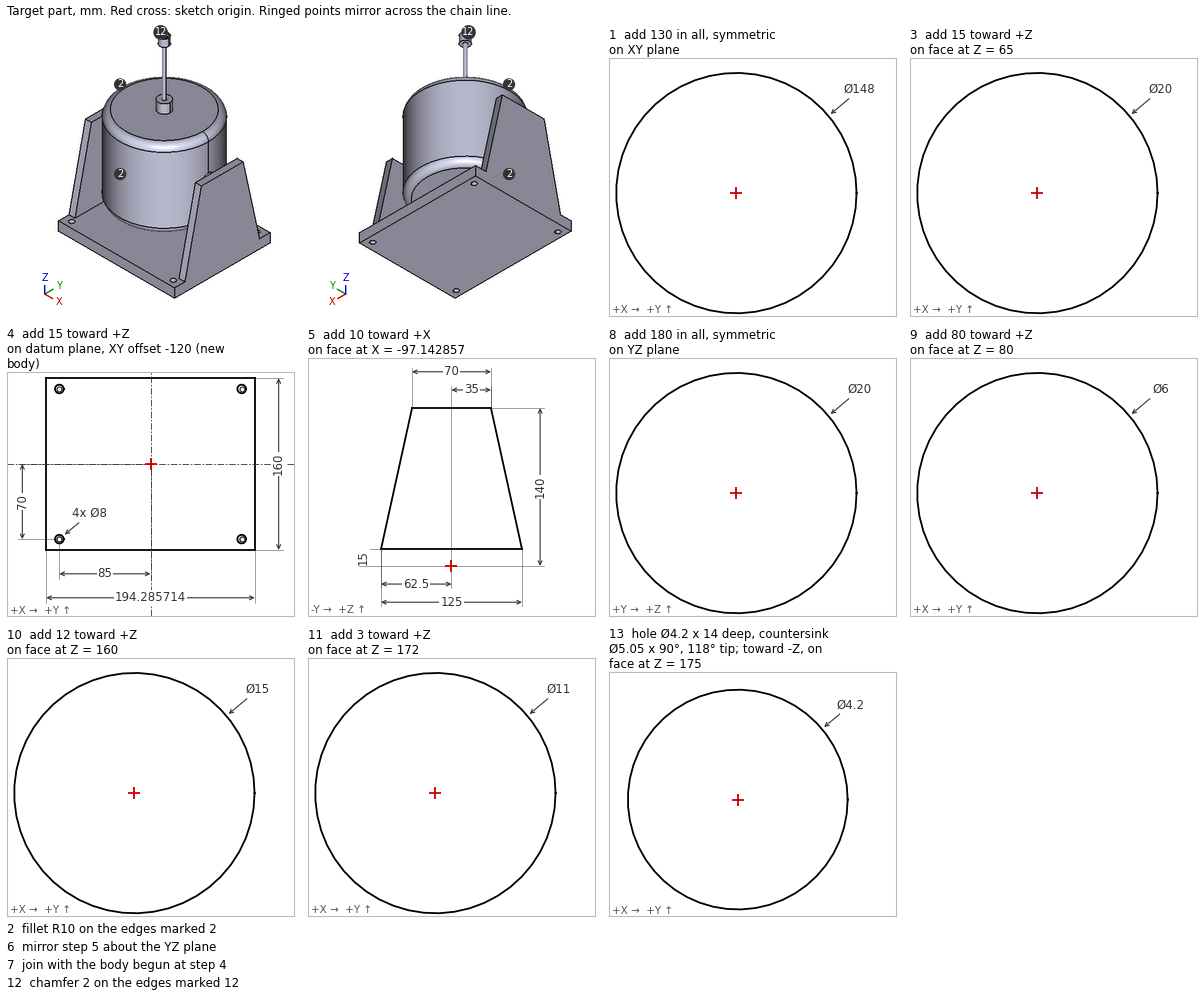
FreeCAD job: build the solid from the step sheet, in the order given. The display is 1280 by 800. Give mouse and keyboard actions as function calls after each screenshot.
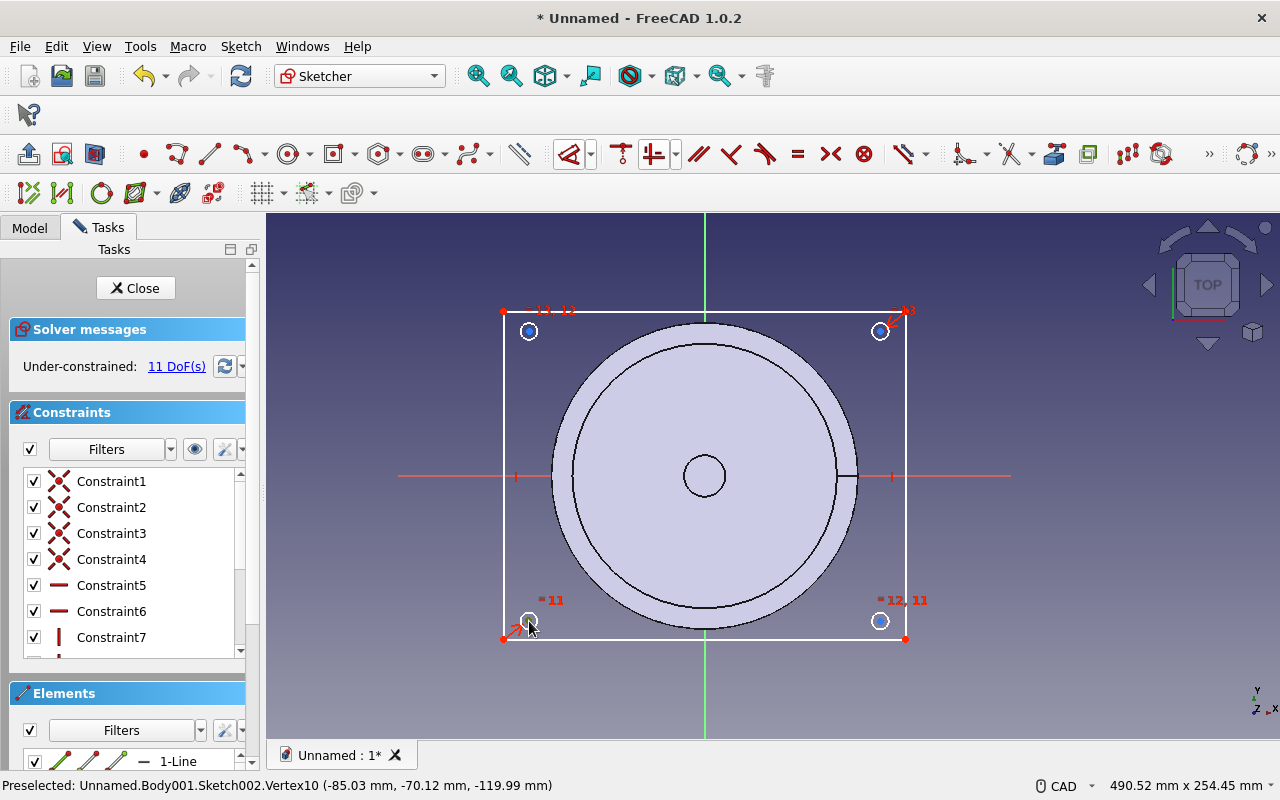
click(880, 621)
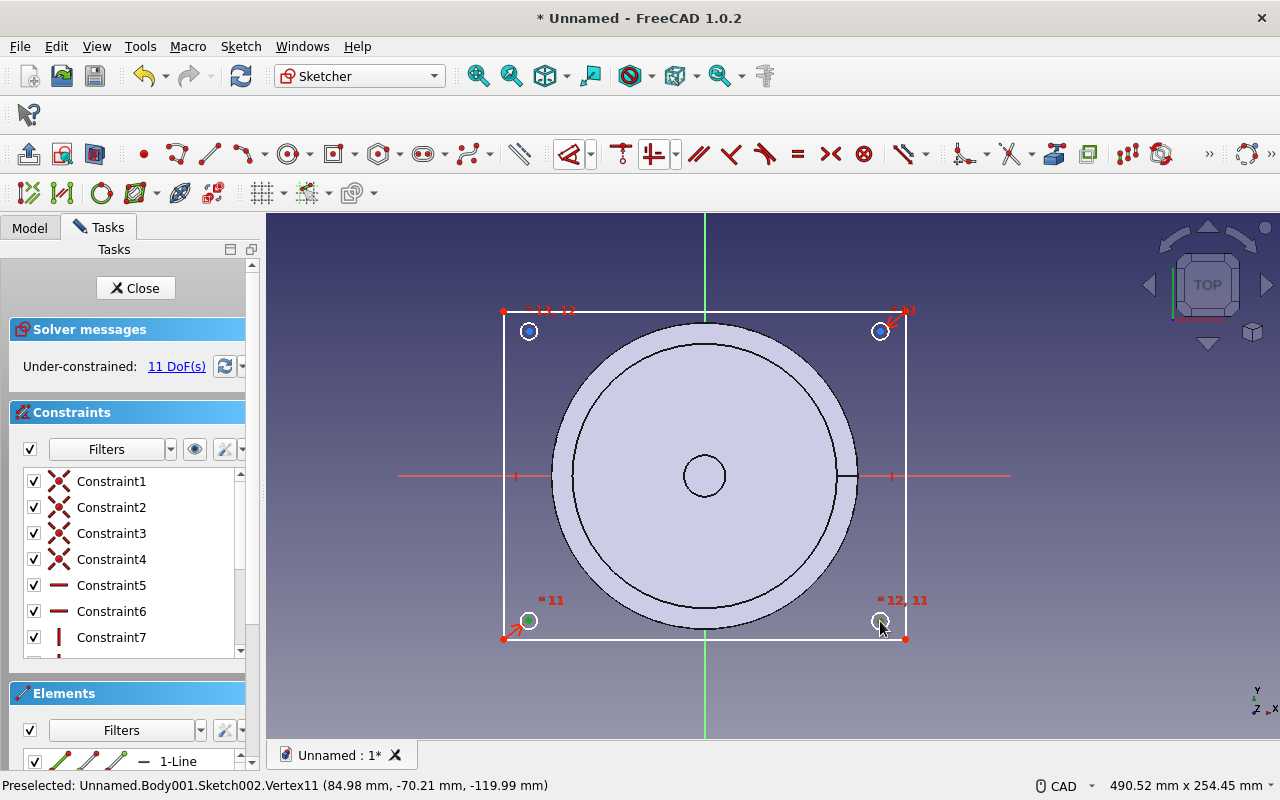
click(705, 677)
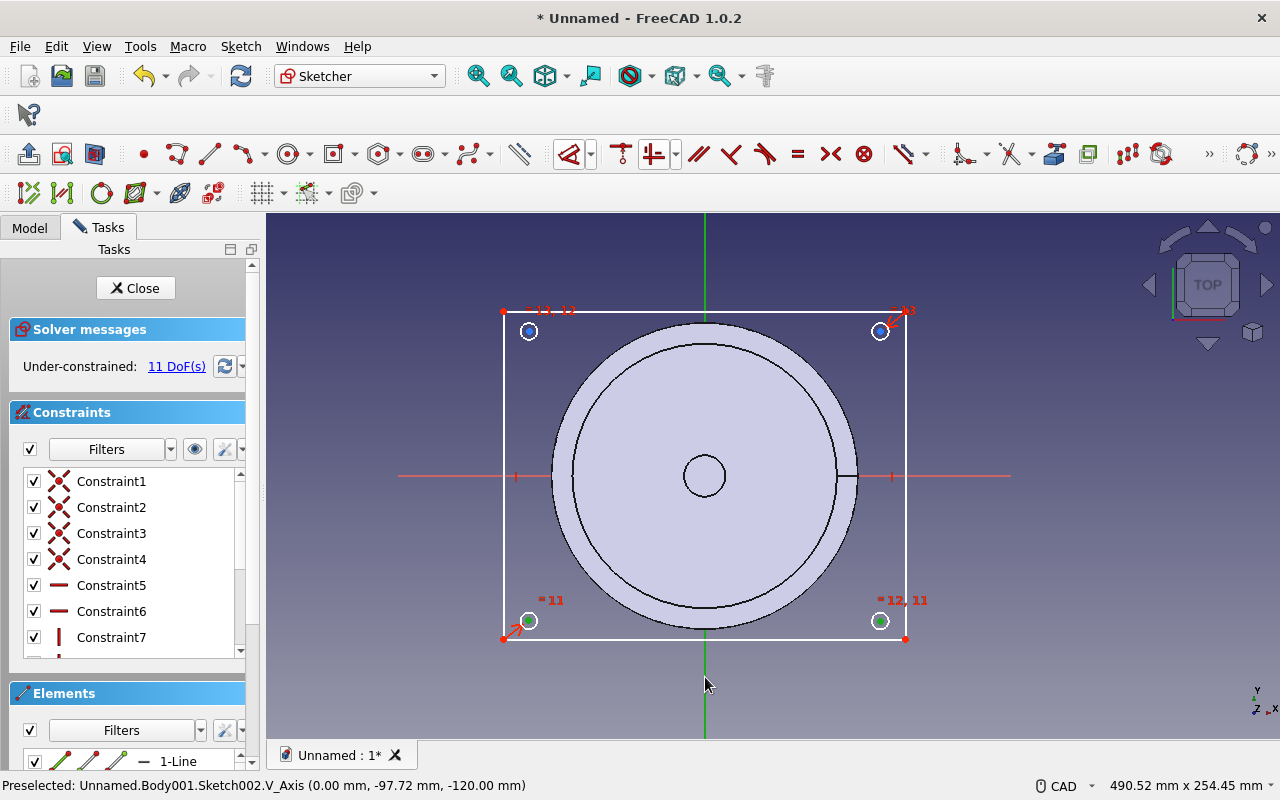
key(s)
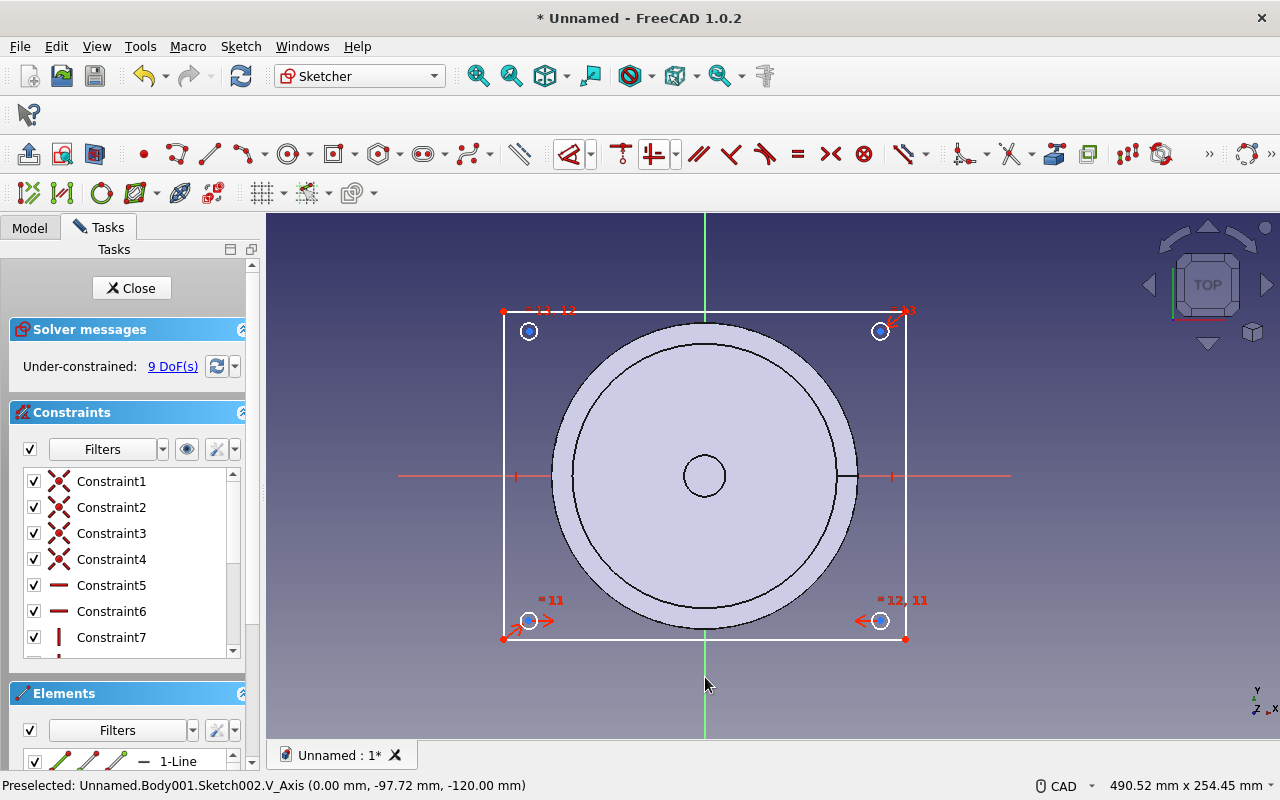
click(529, 621)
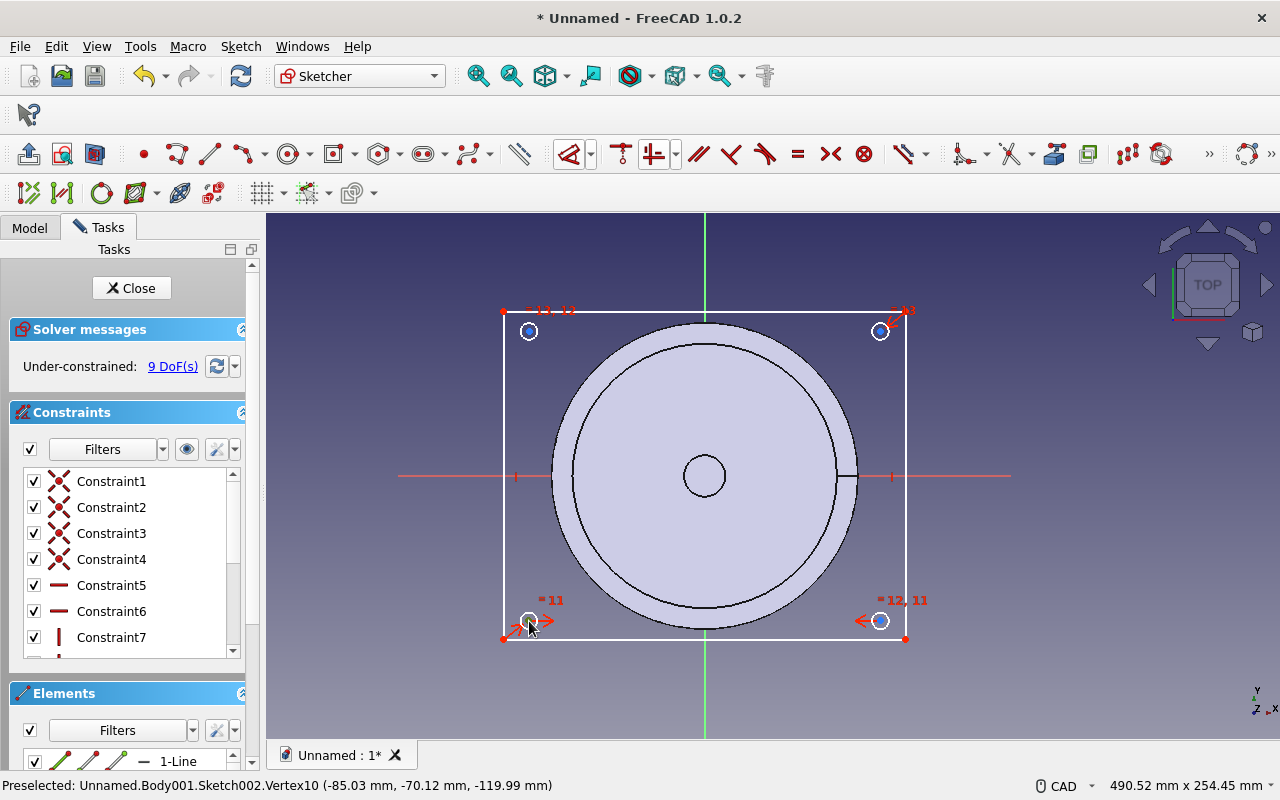
click(529, 331)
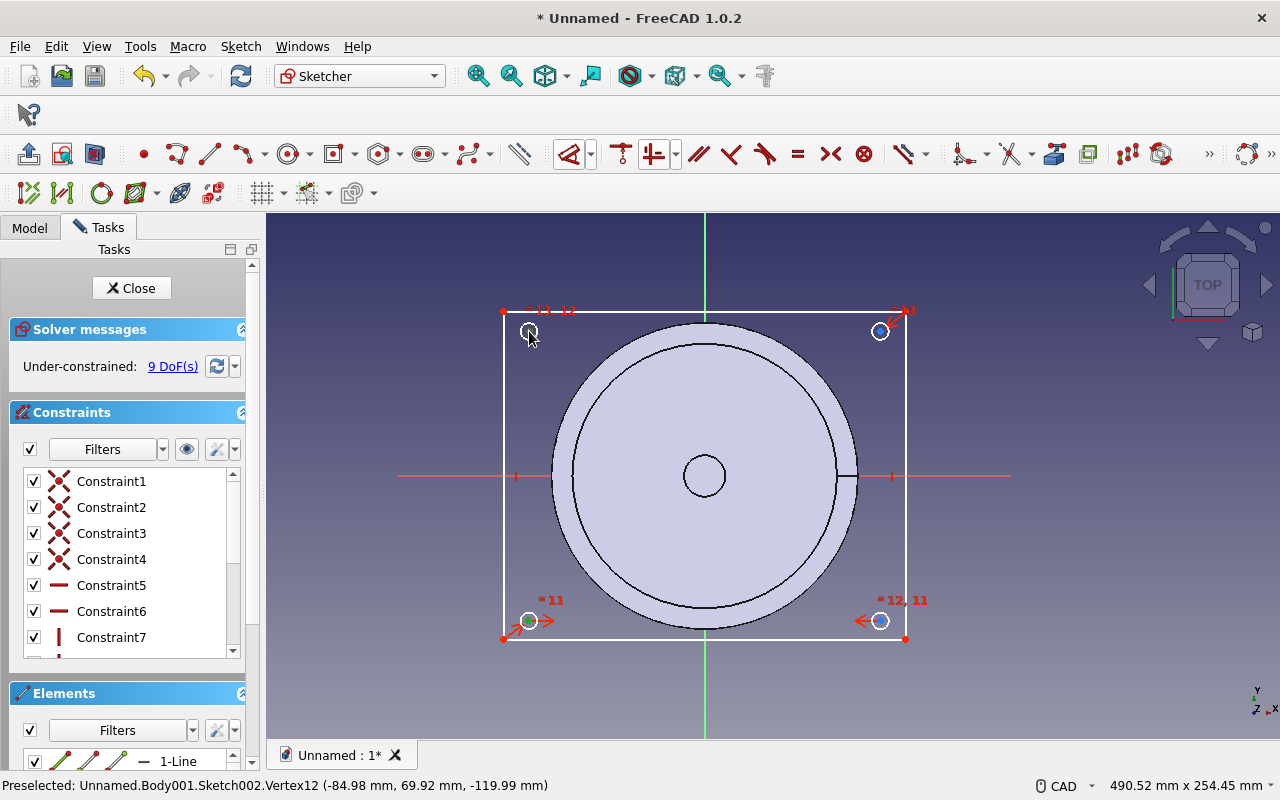
click(411, 476)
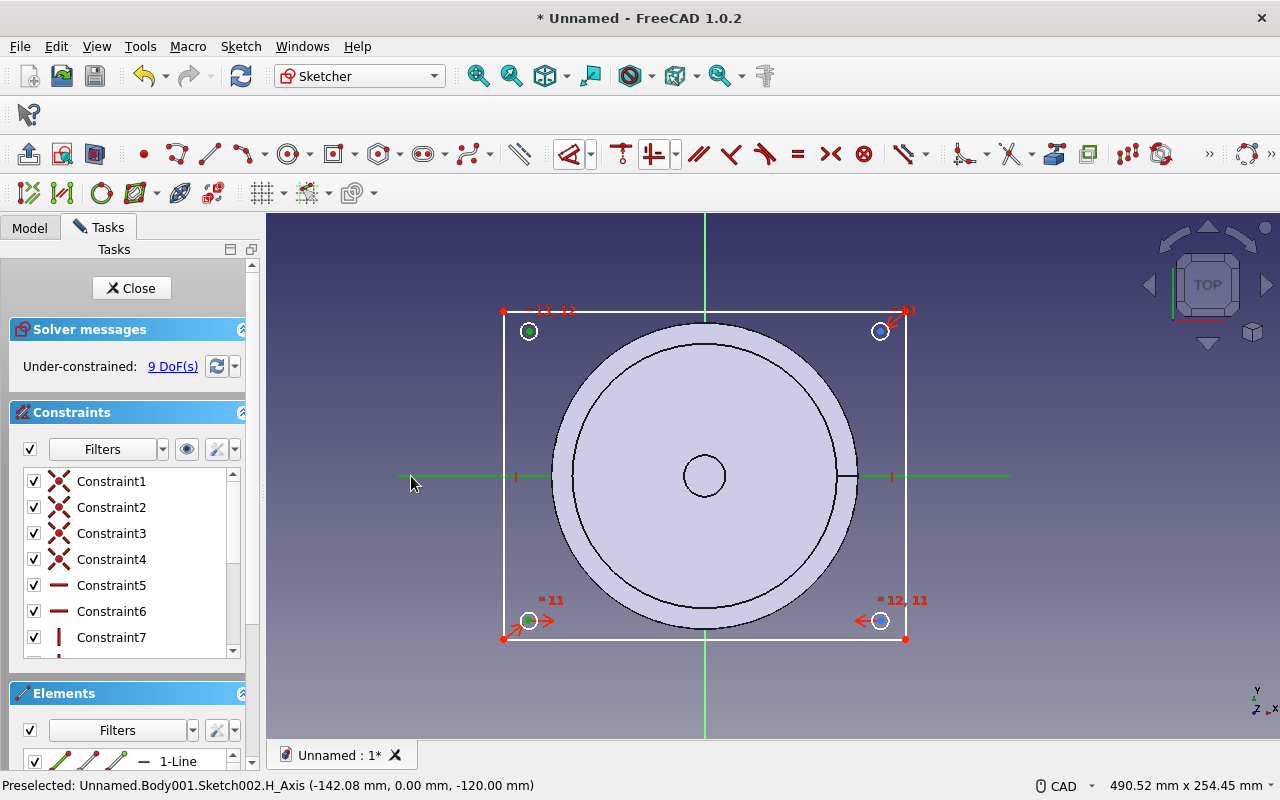
click(831, 154)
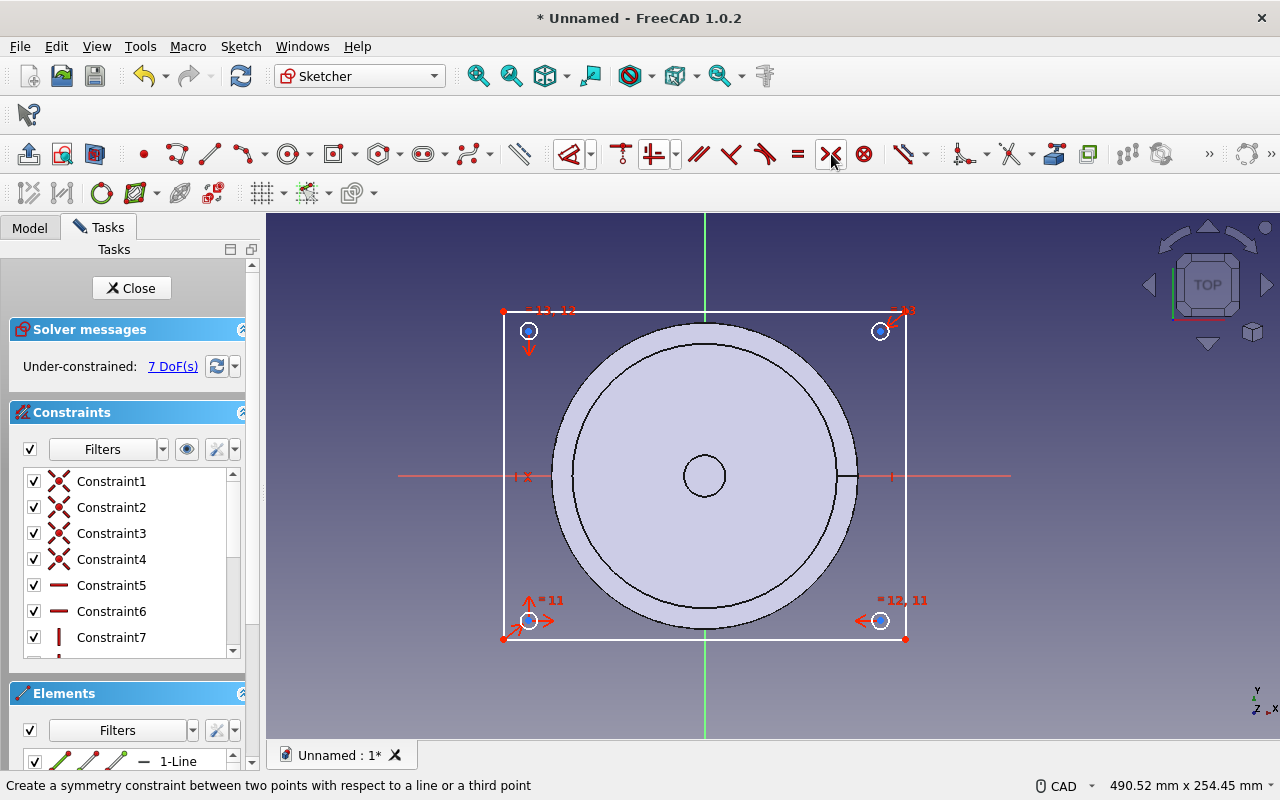
click(880, 621)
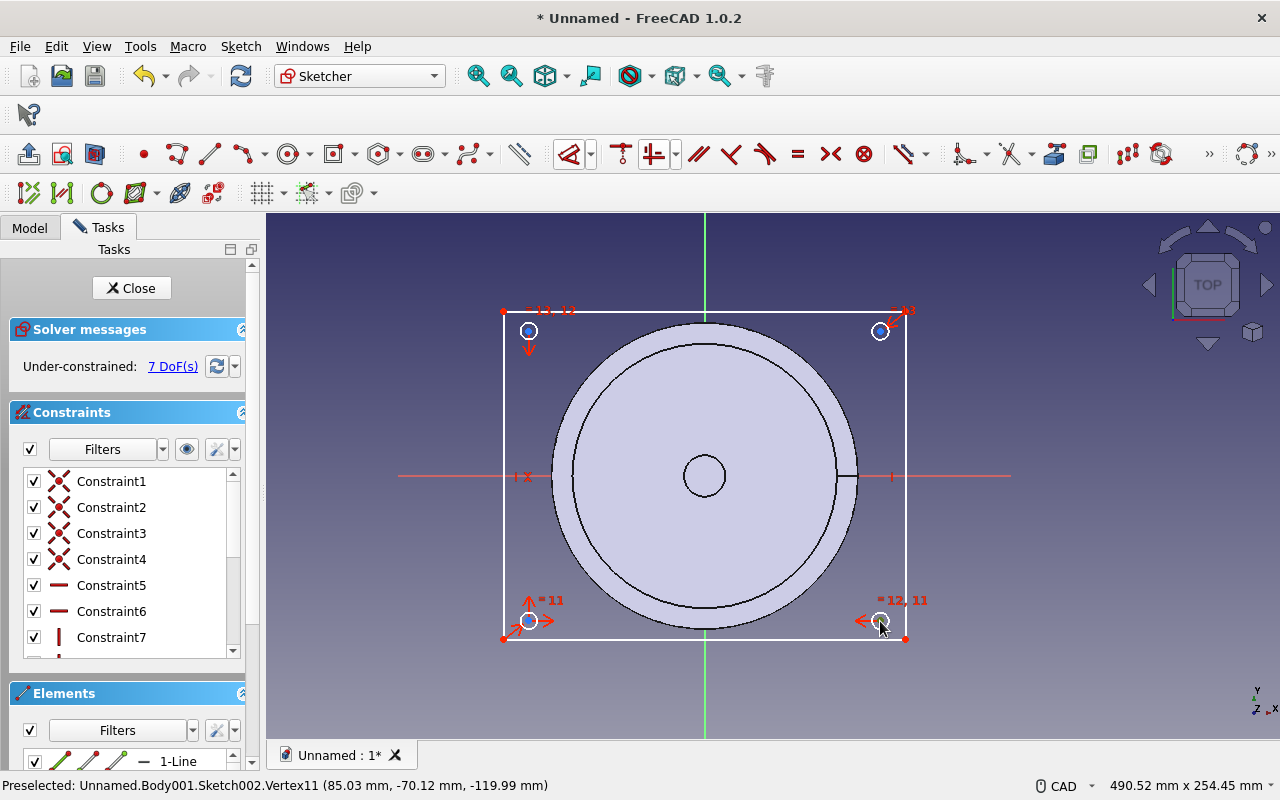
click(880, 331)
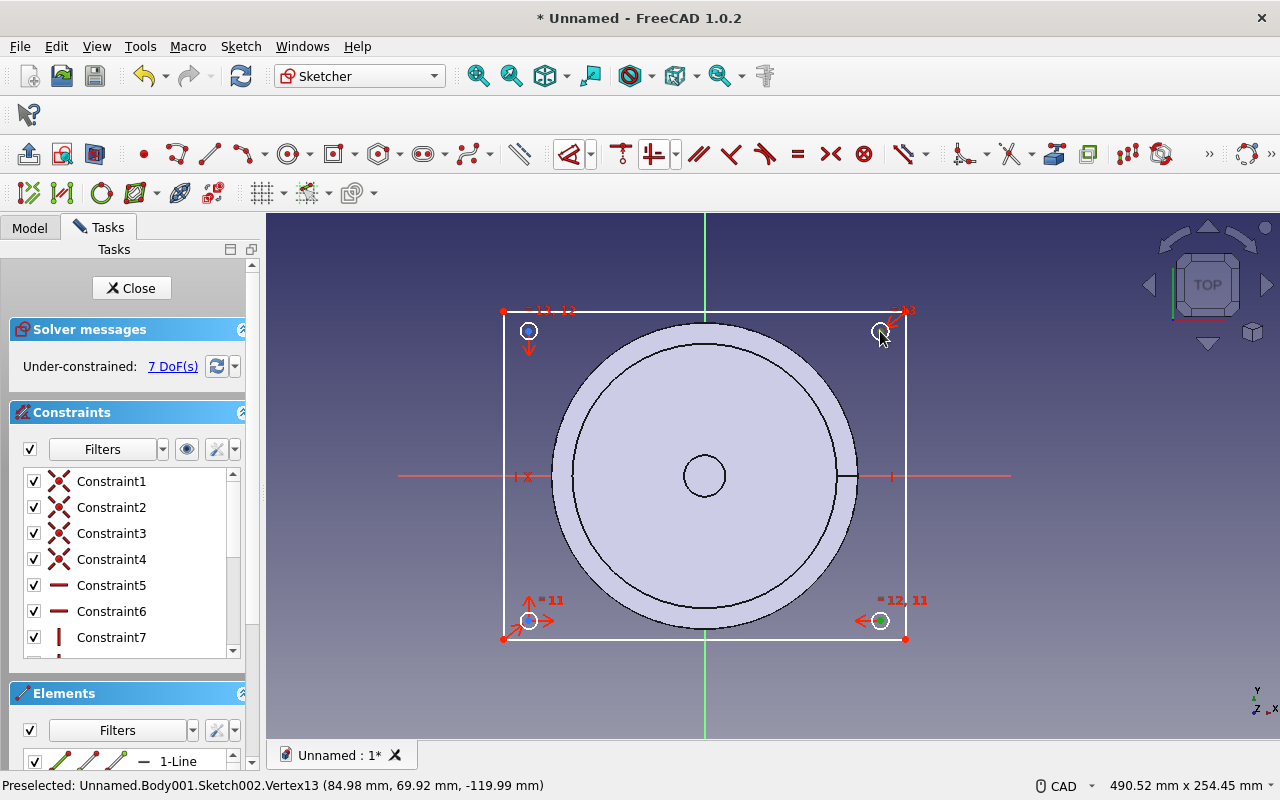
click(411, 476)